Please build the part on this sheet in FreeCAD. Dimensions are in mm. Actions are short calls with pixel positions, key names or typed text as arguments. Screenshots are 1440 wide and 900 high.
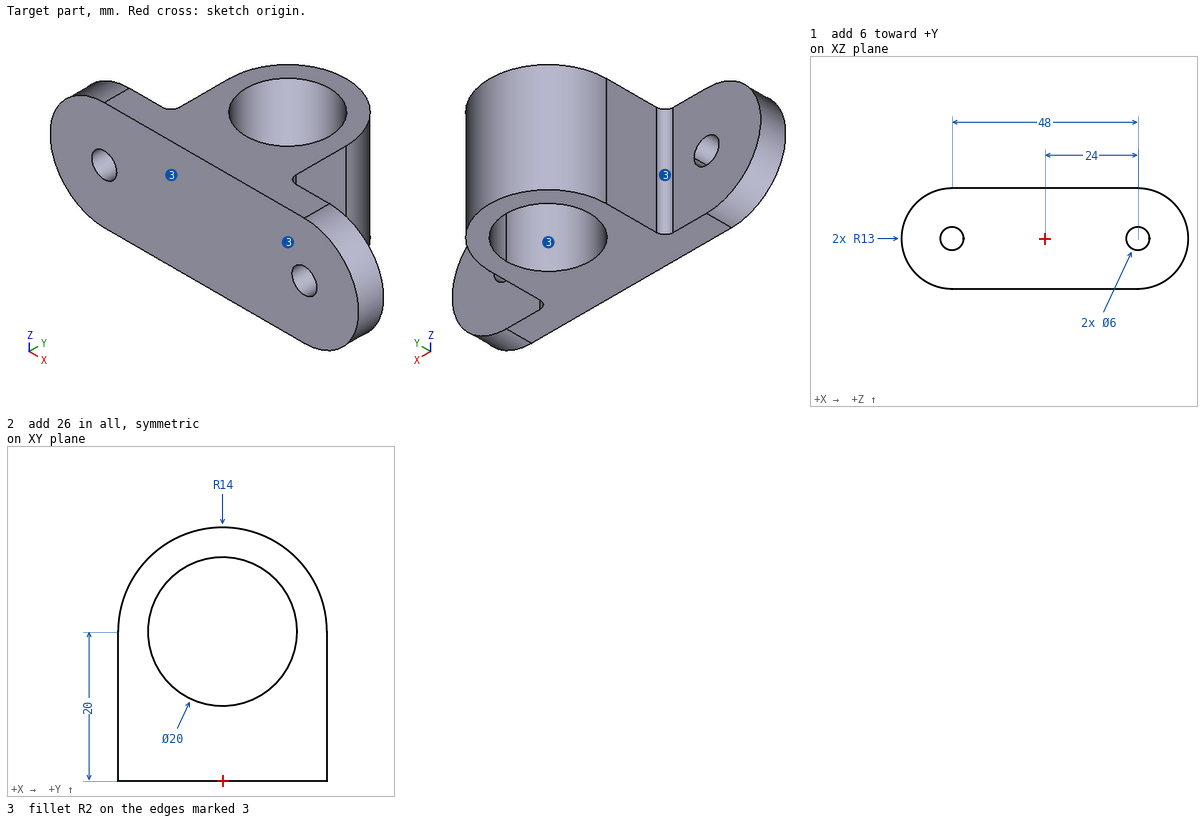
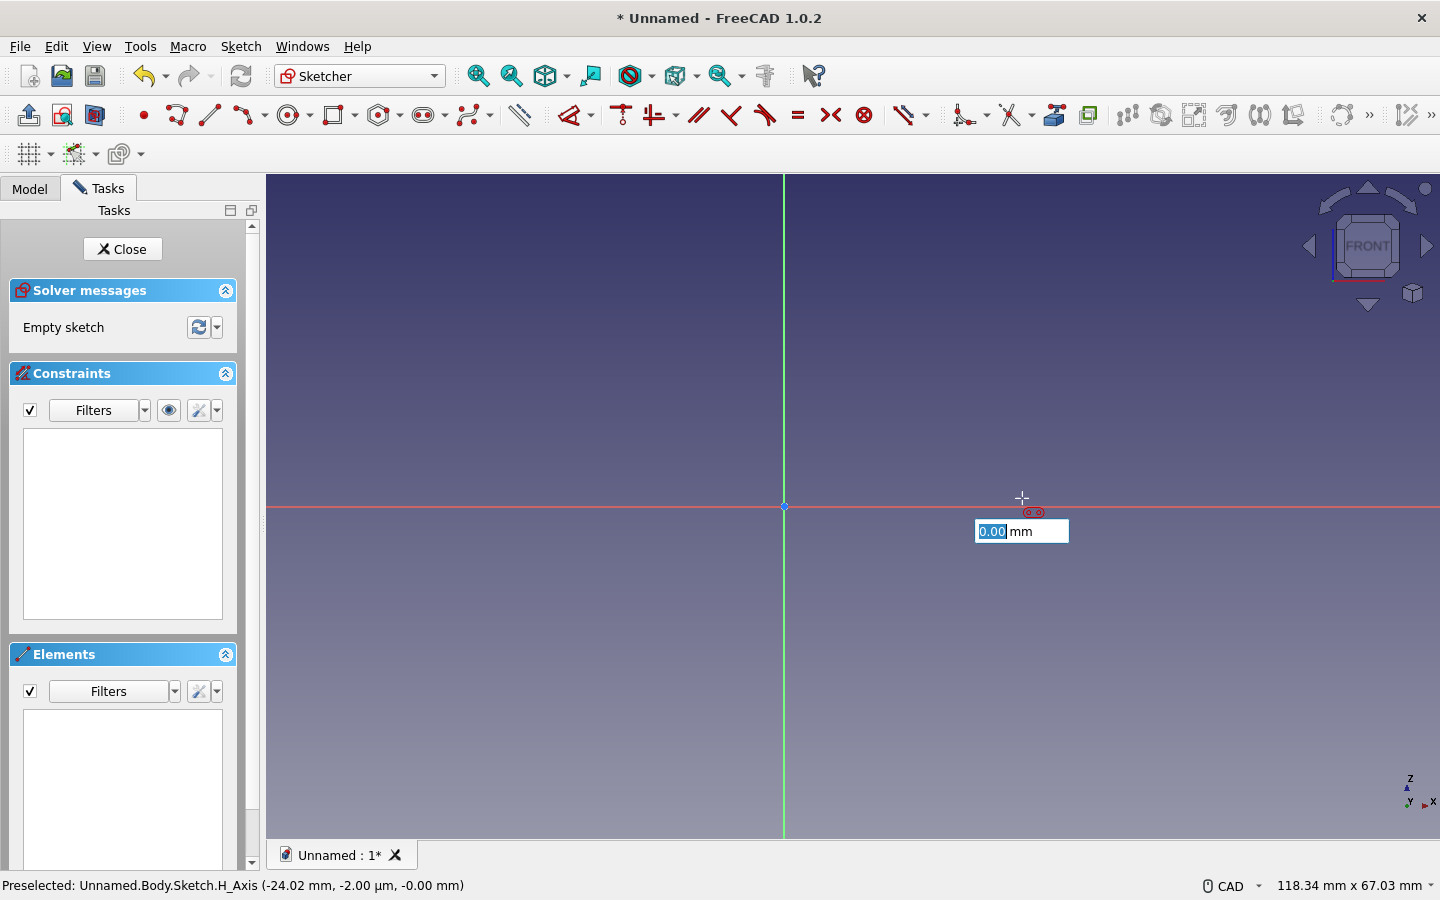
click(856, 635)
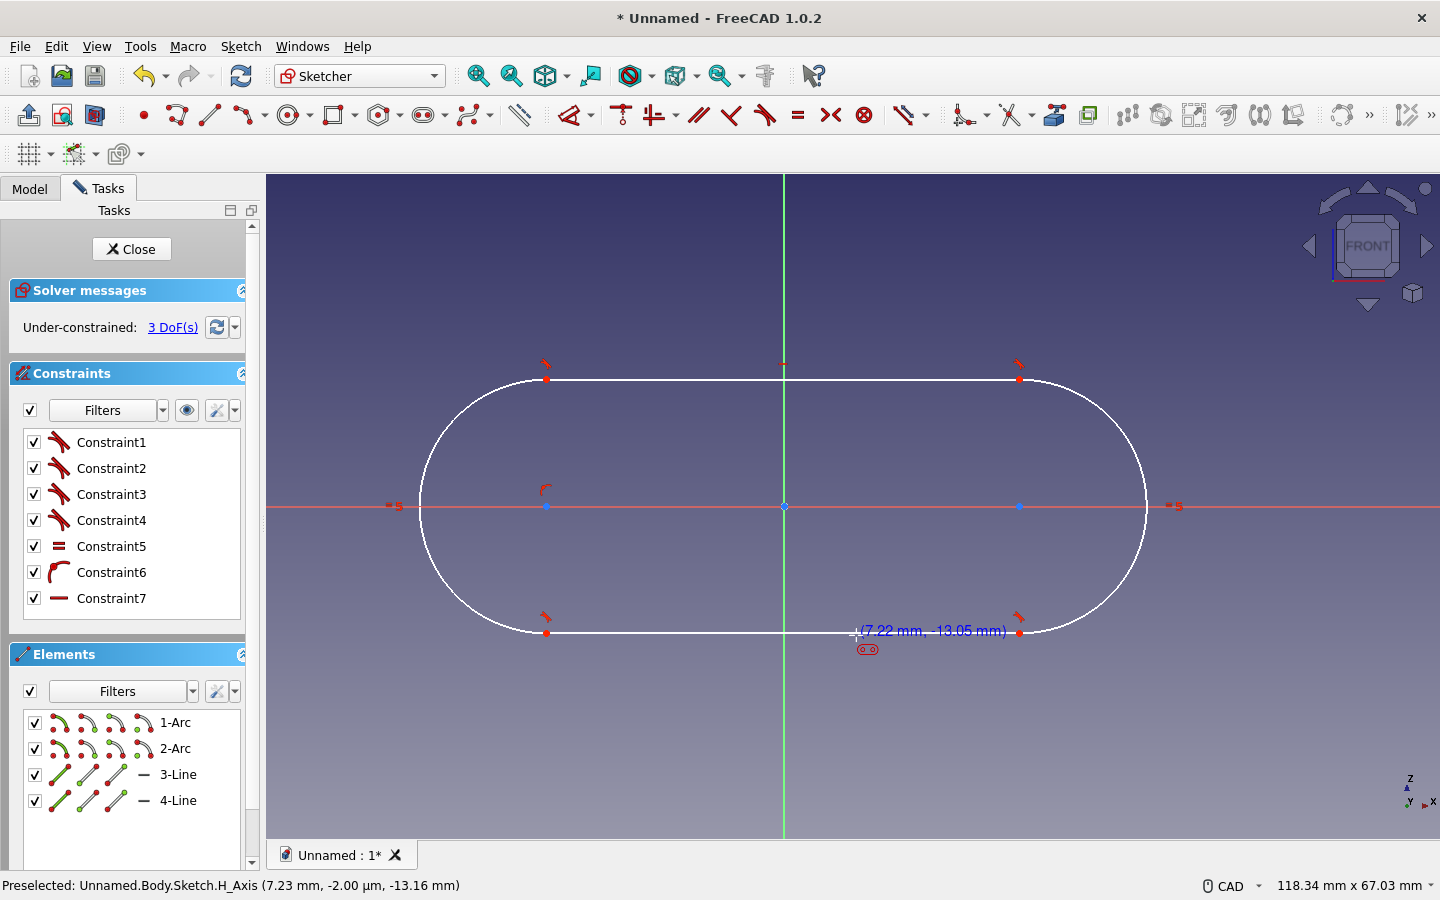
key(g)
key(c)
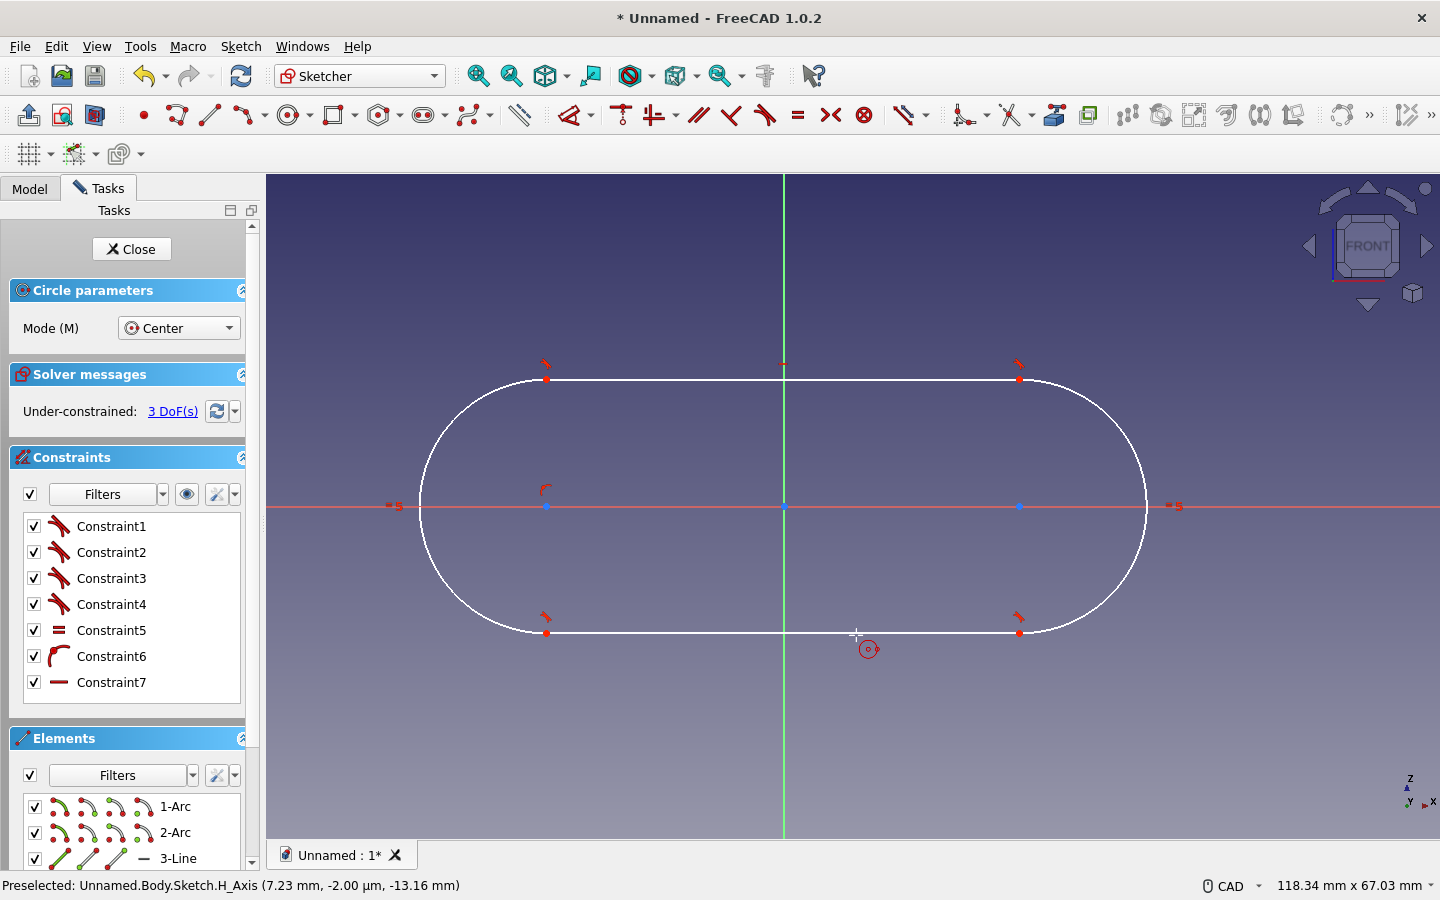
click(1020, 506)
click(1043, 485)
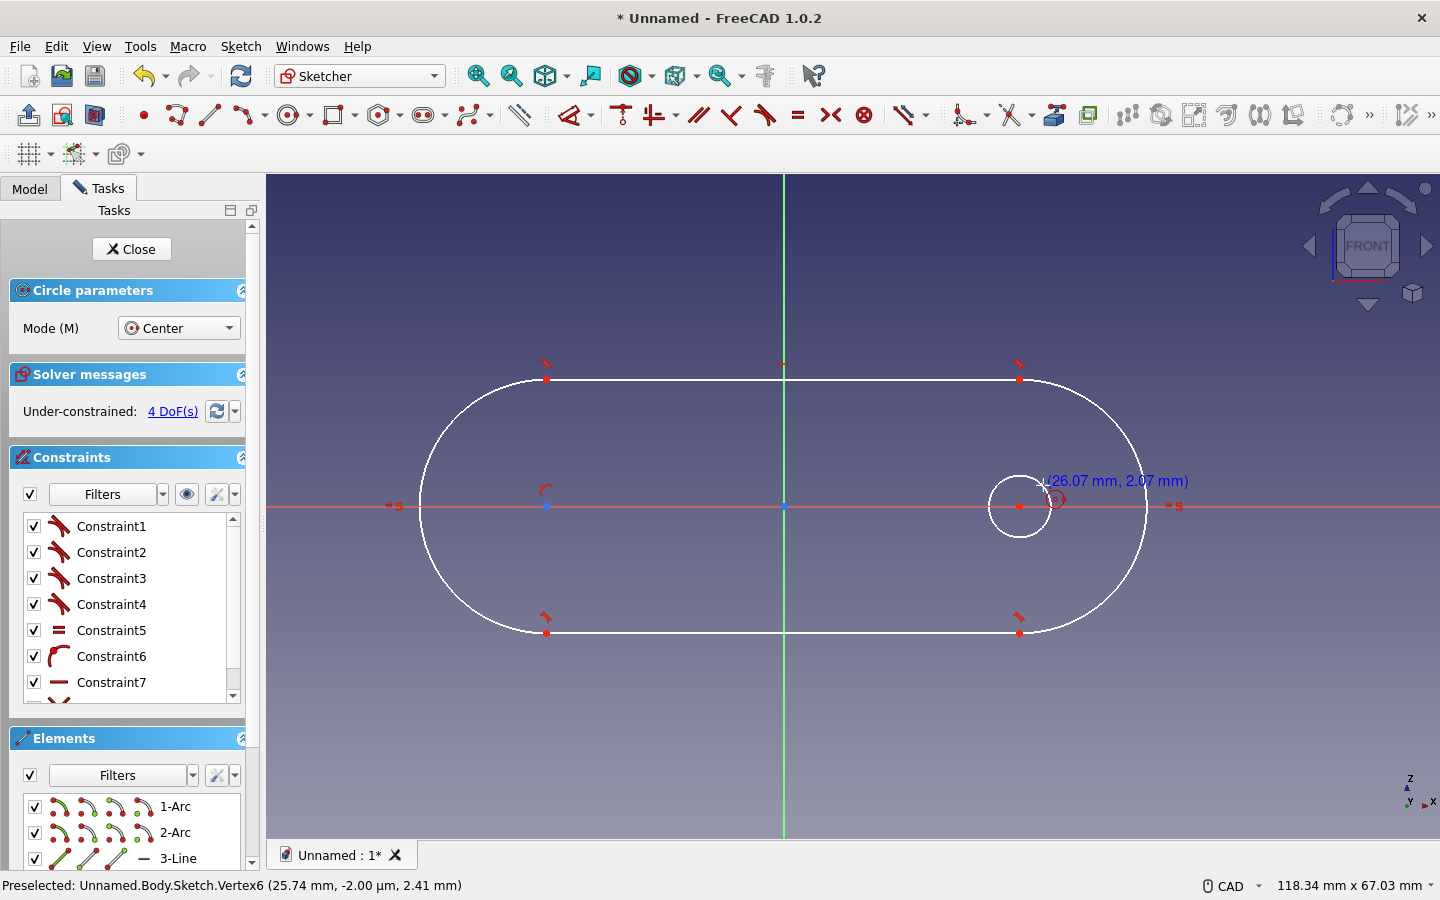
click(546, 506)
click(567, 485)
key(Escape)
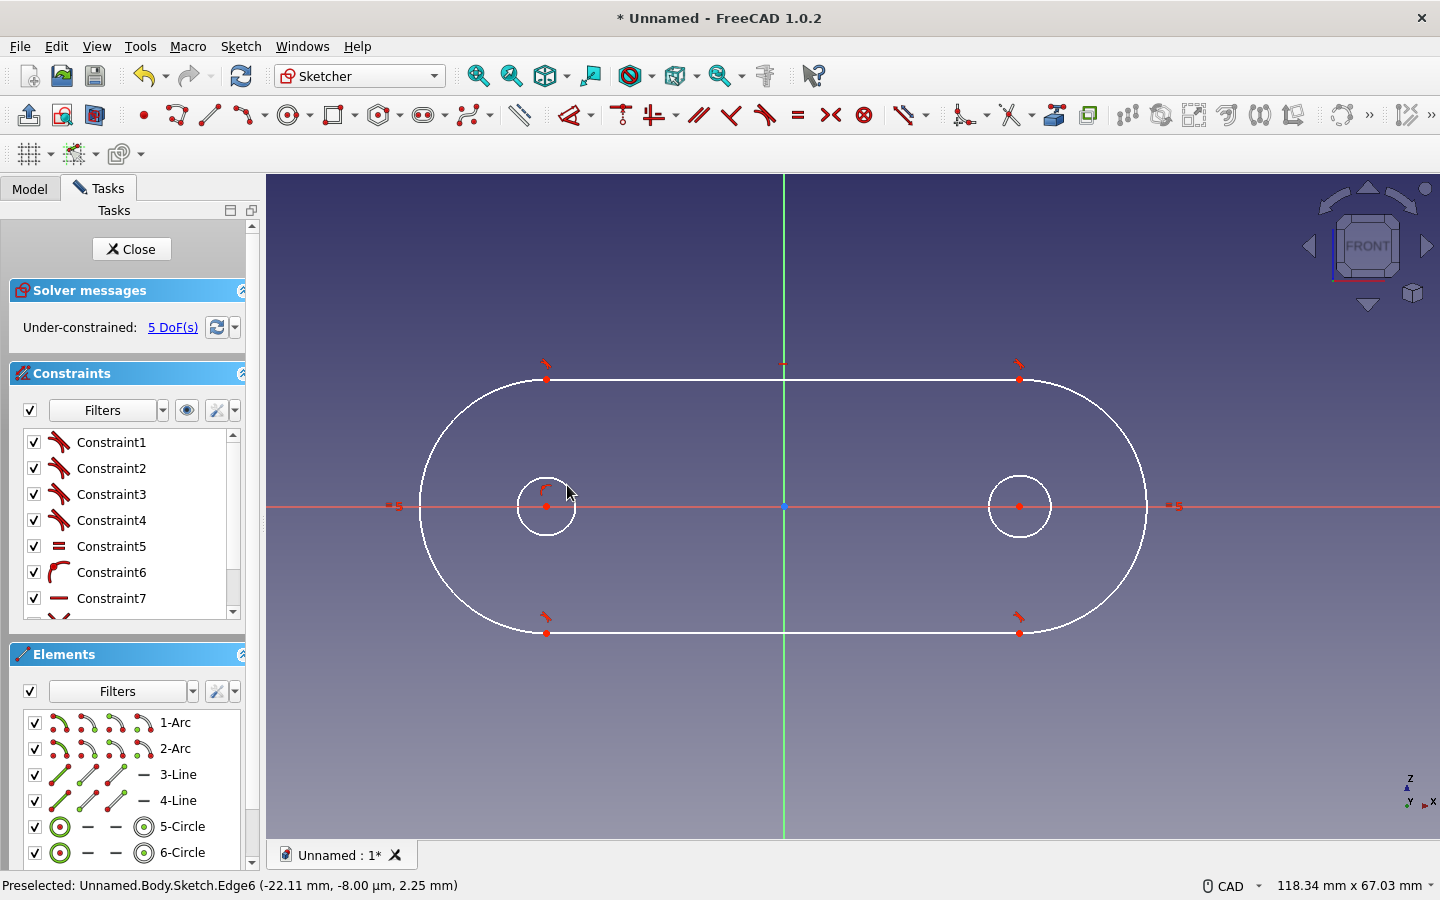
click(1042, 485)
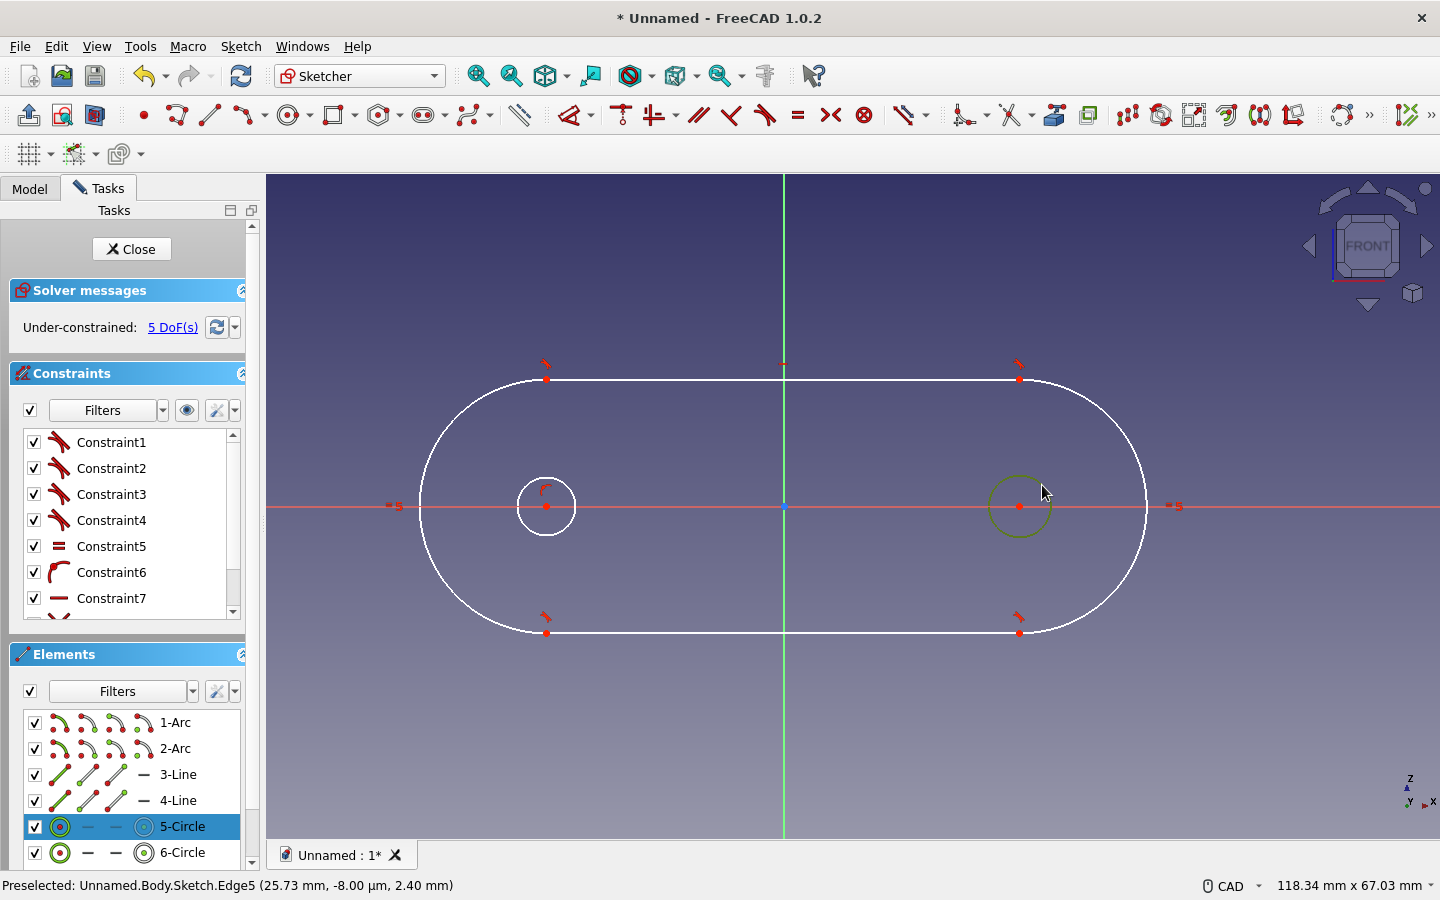
click(567, 486)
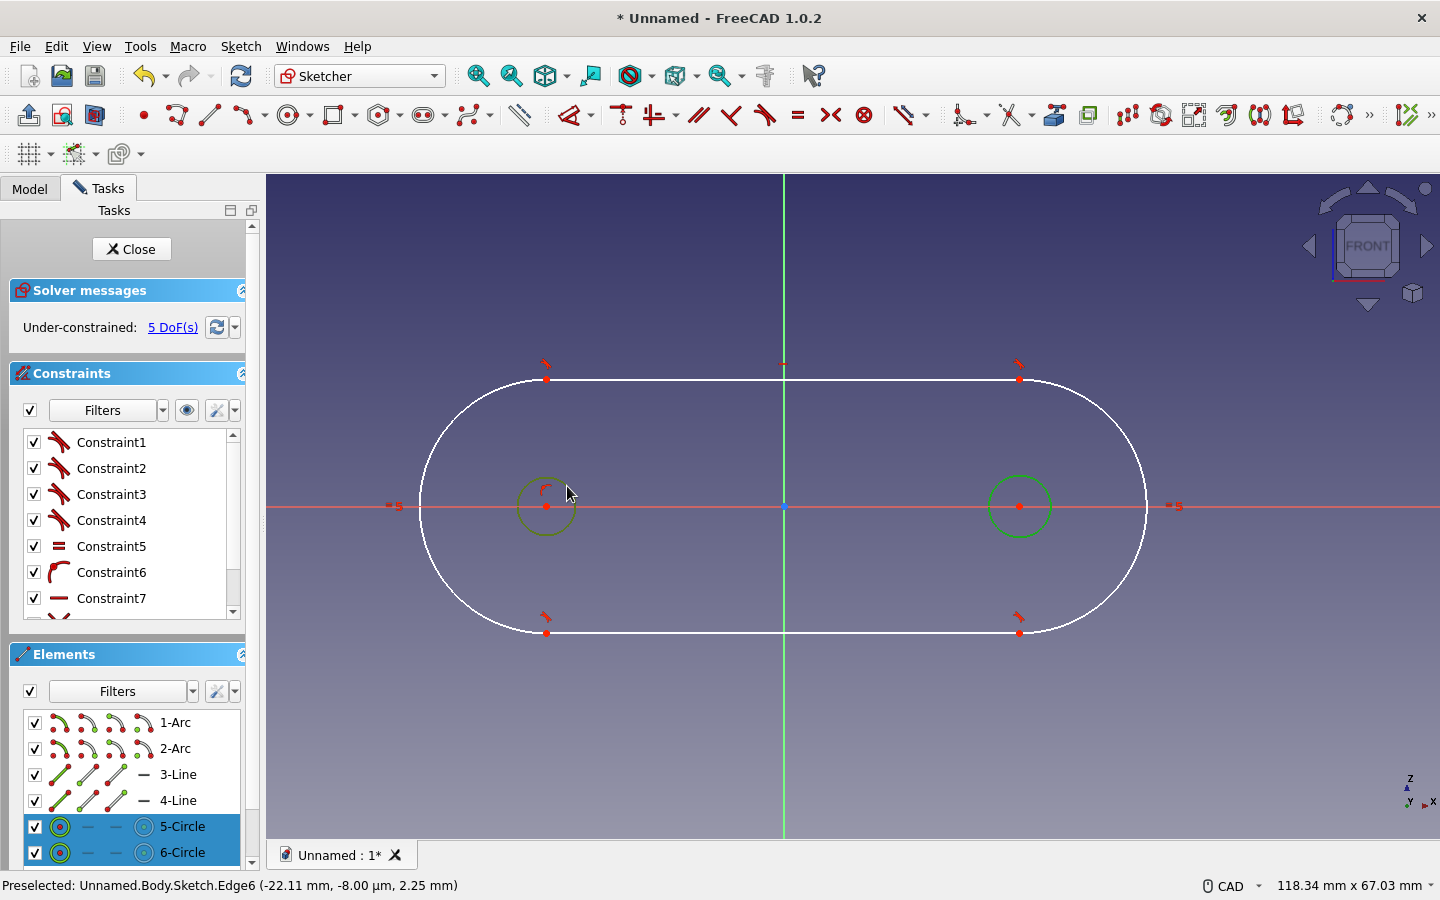
key(e)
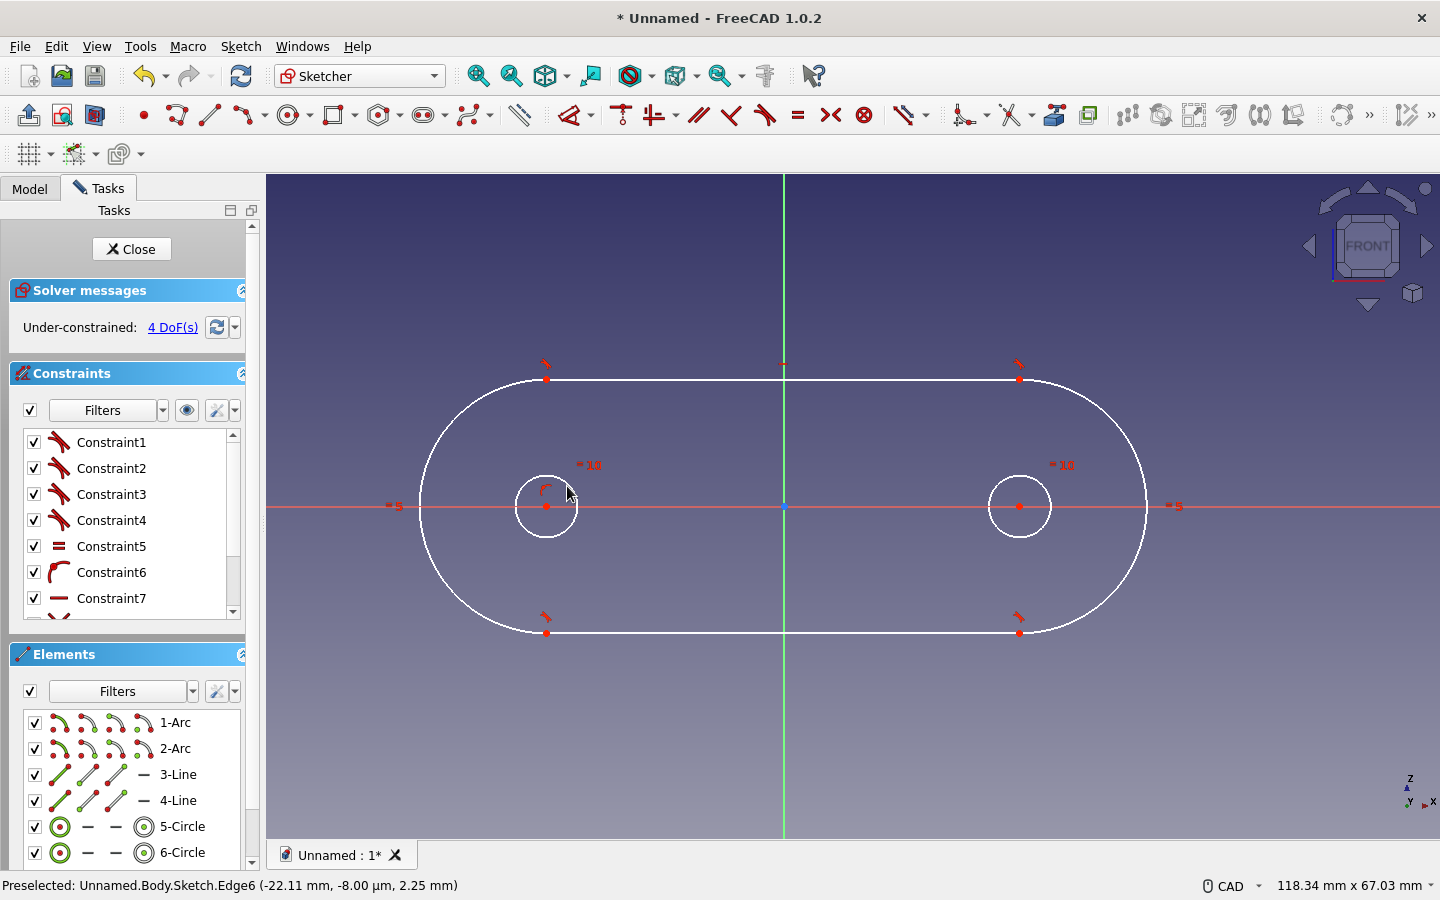
click(444, 432)